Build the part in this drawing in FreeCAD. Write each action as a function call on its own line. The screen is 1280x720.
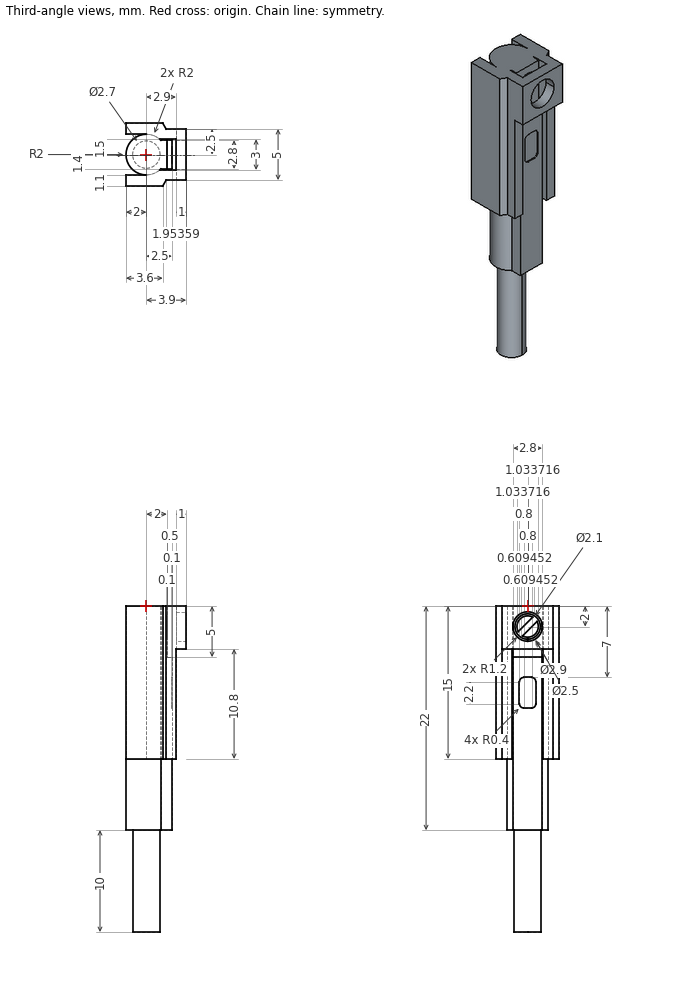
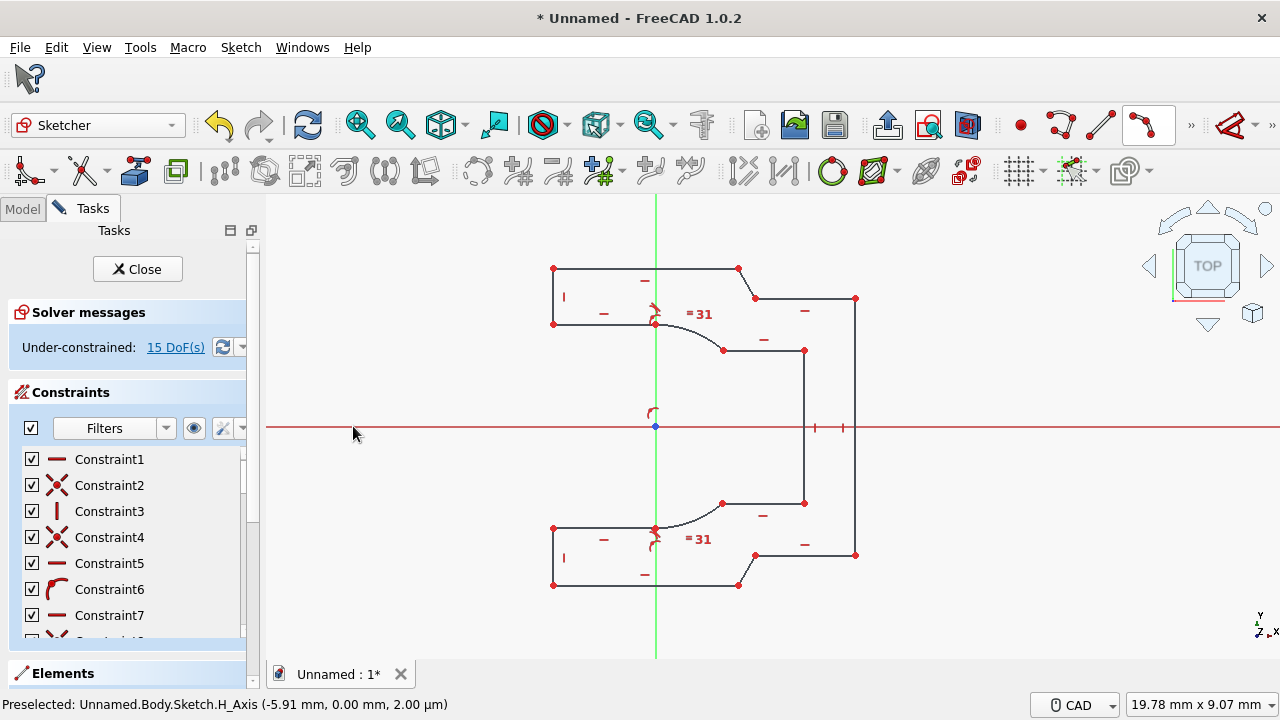
click(755, 556)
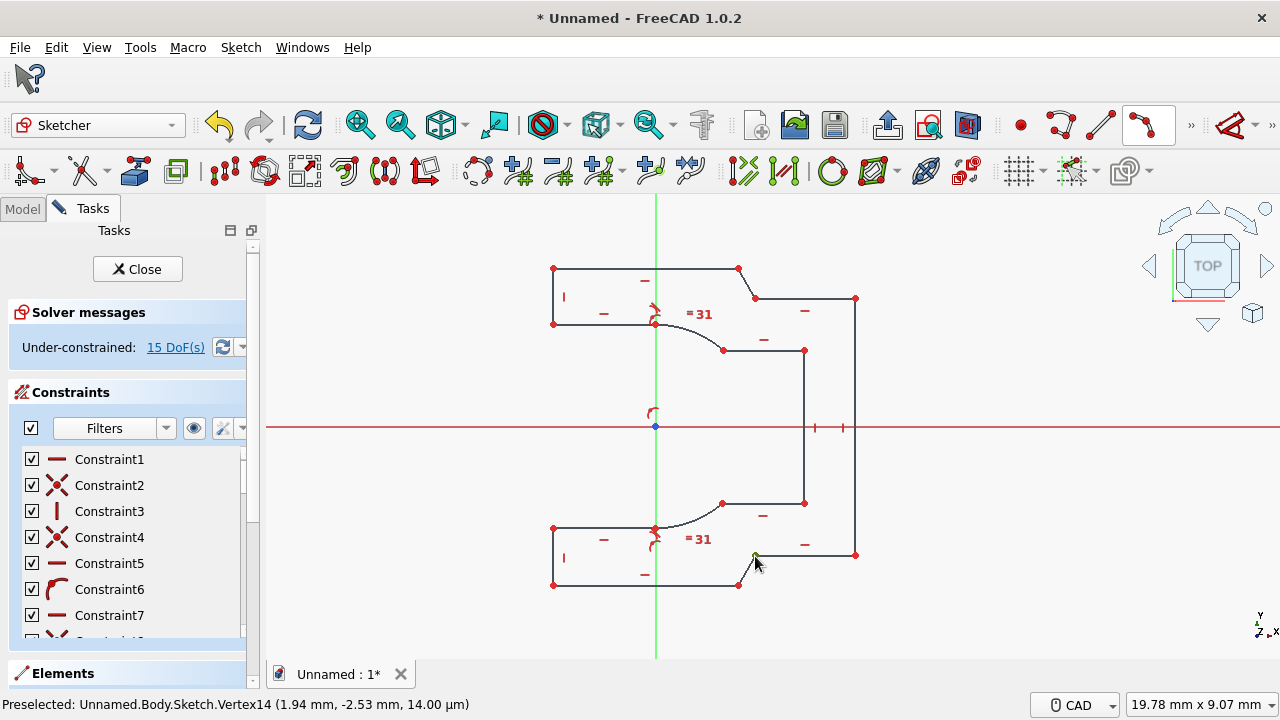
click(755, 299)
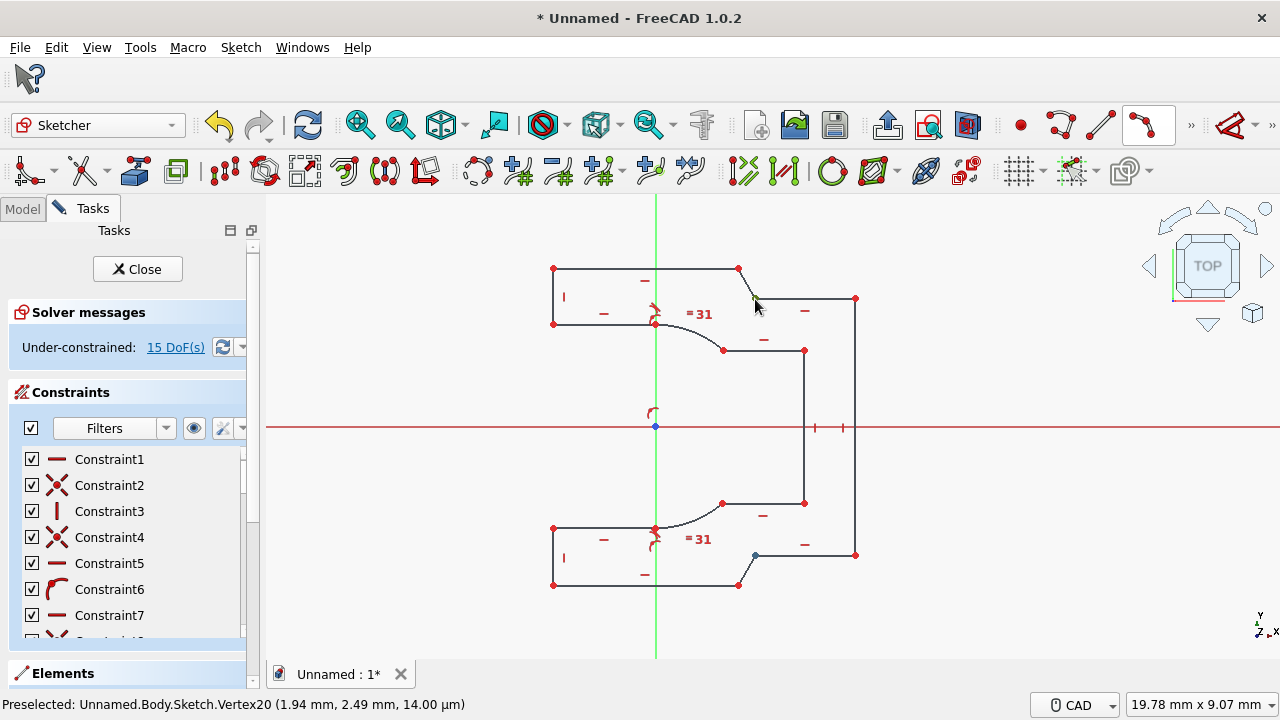
click(353, 426)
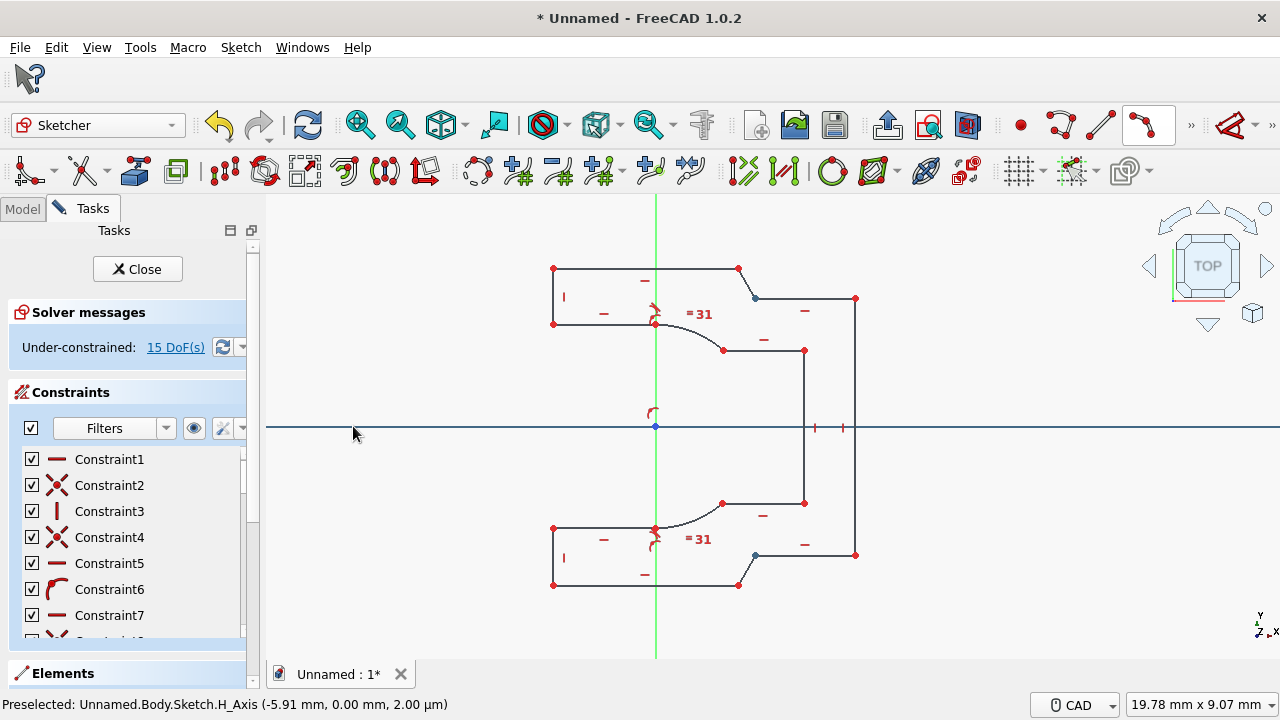
key(s)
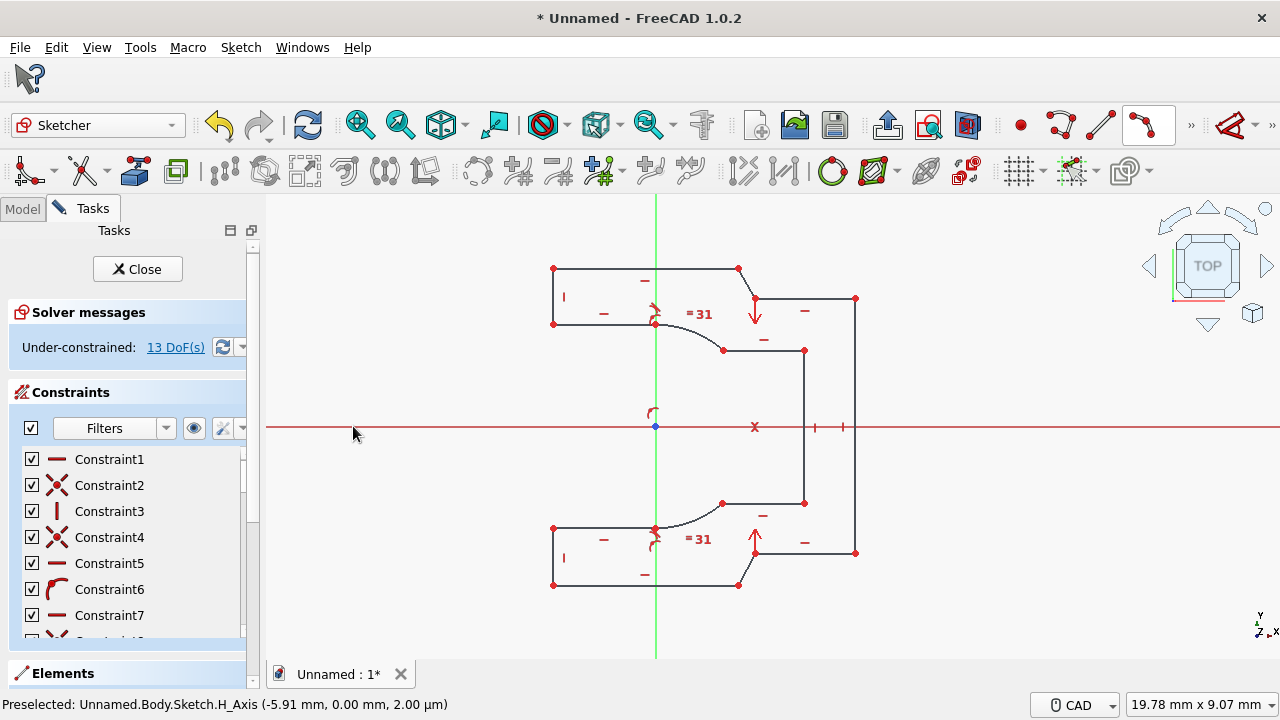
click(738, 586)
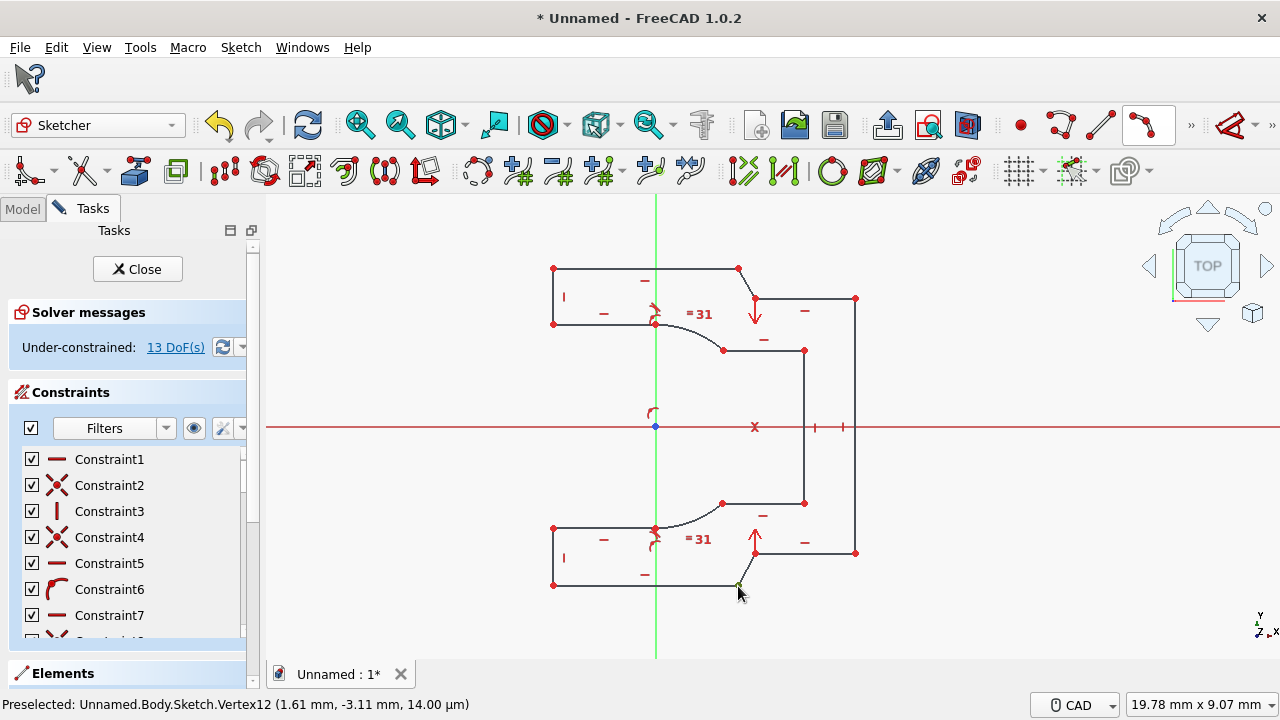
click(738, 269)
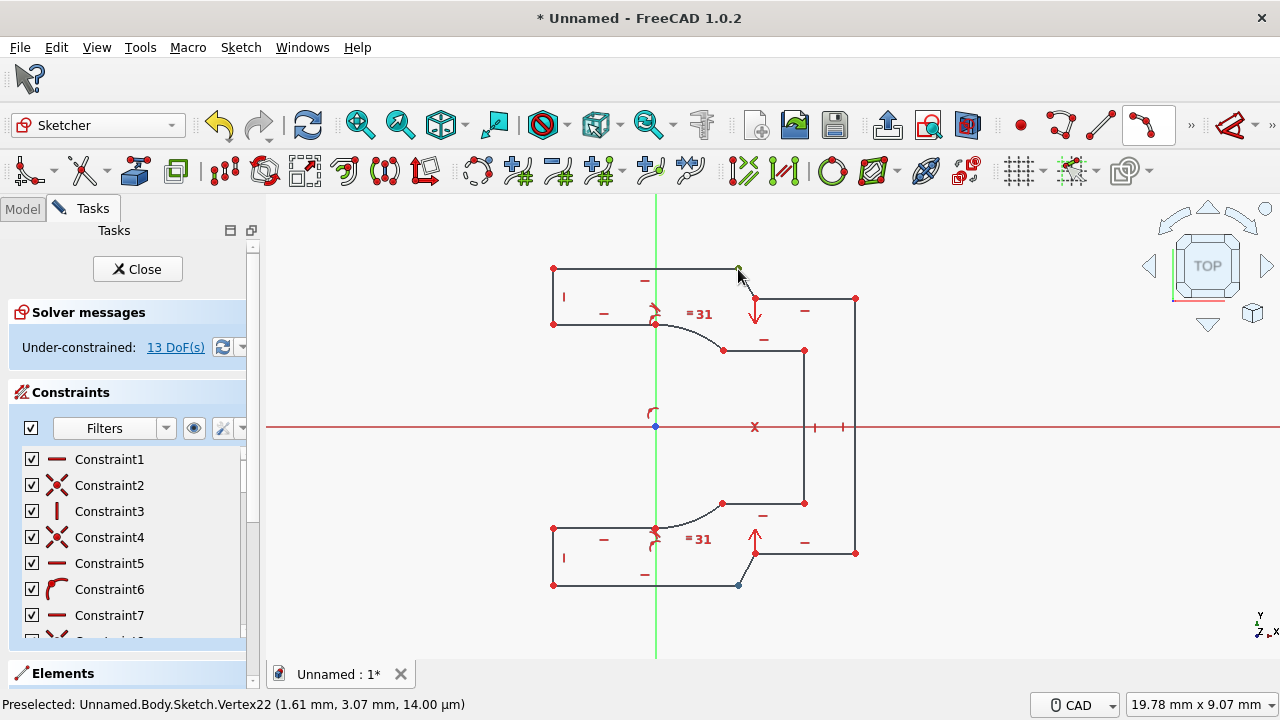
click(353, 426)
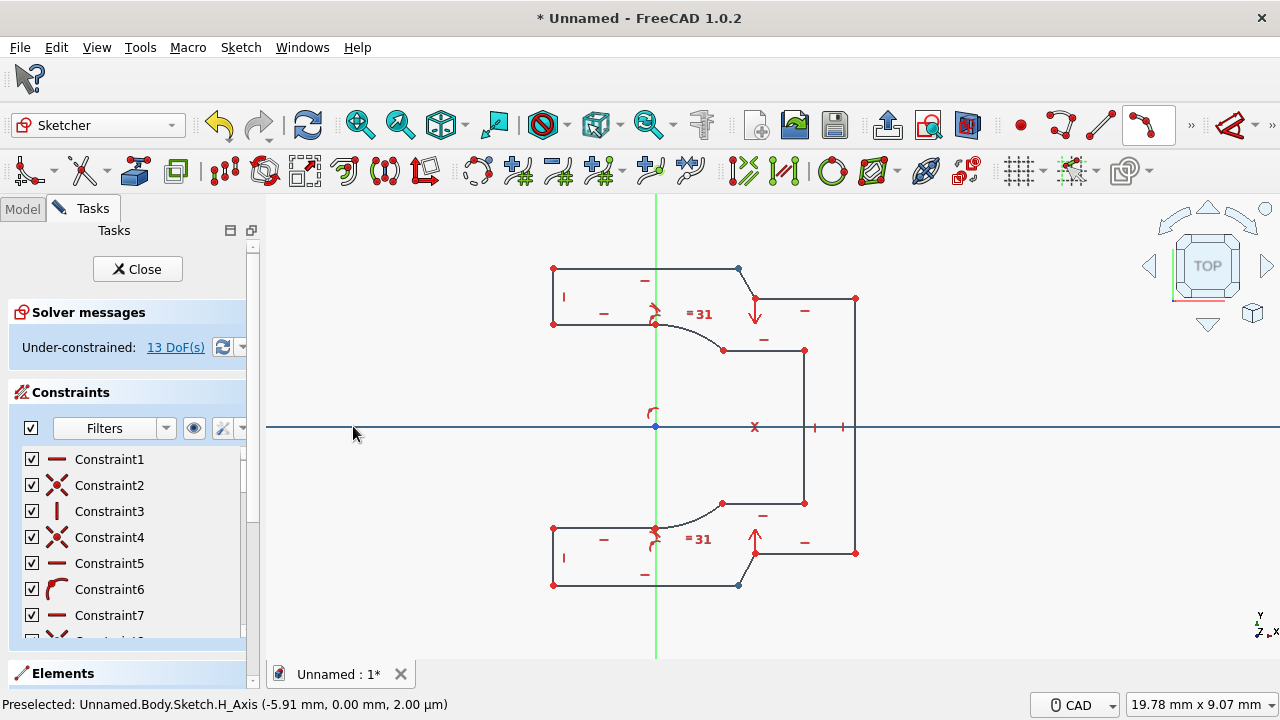
key(s)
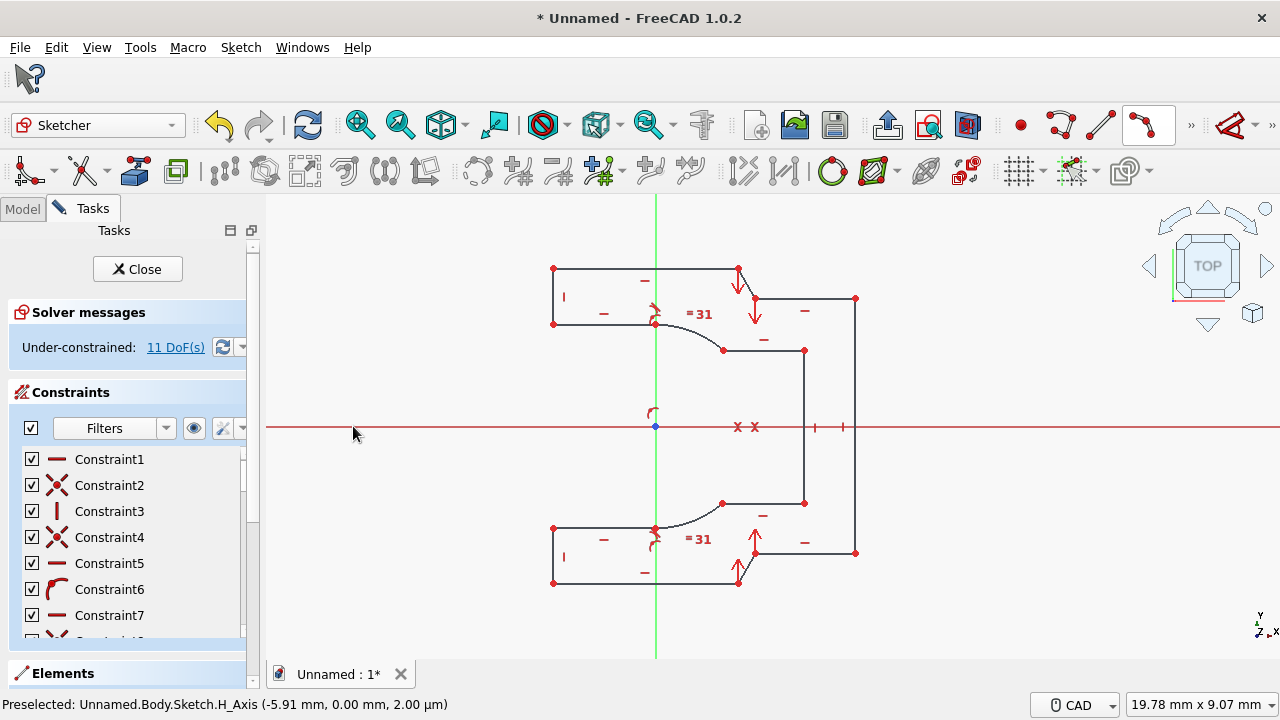
click(1230, 126)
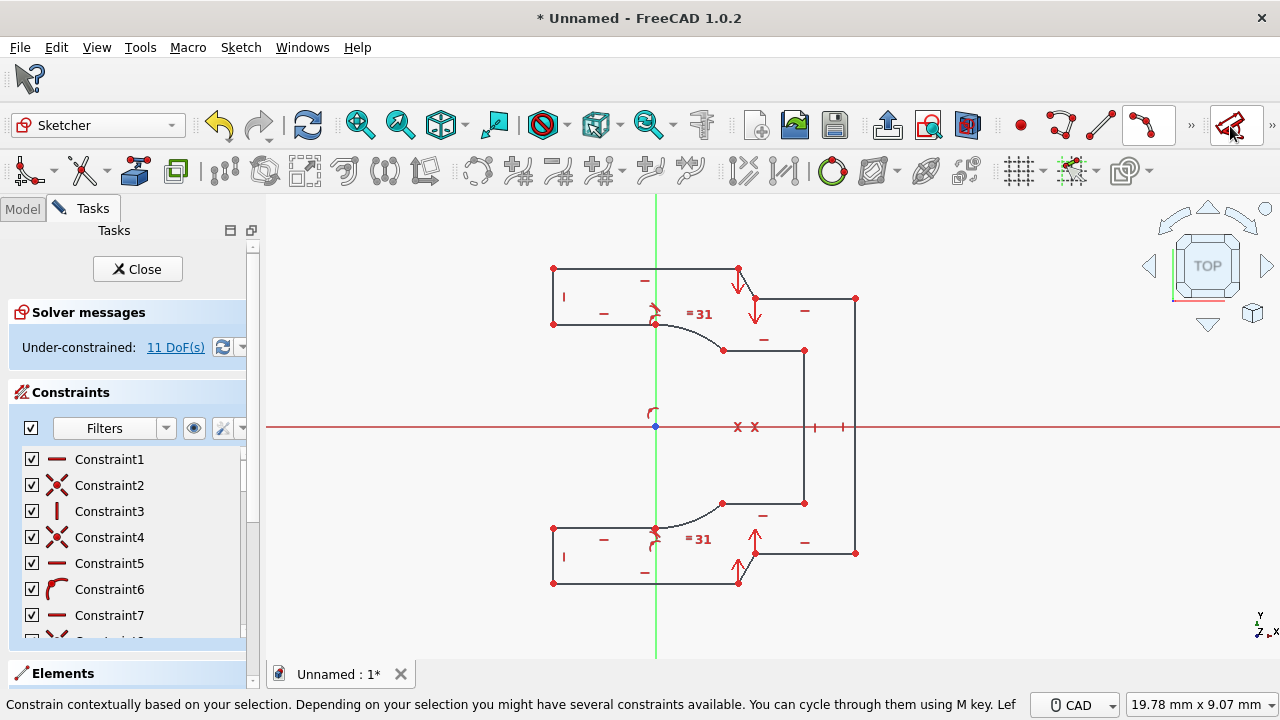
click(677, 526)
click(684, 557)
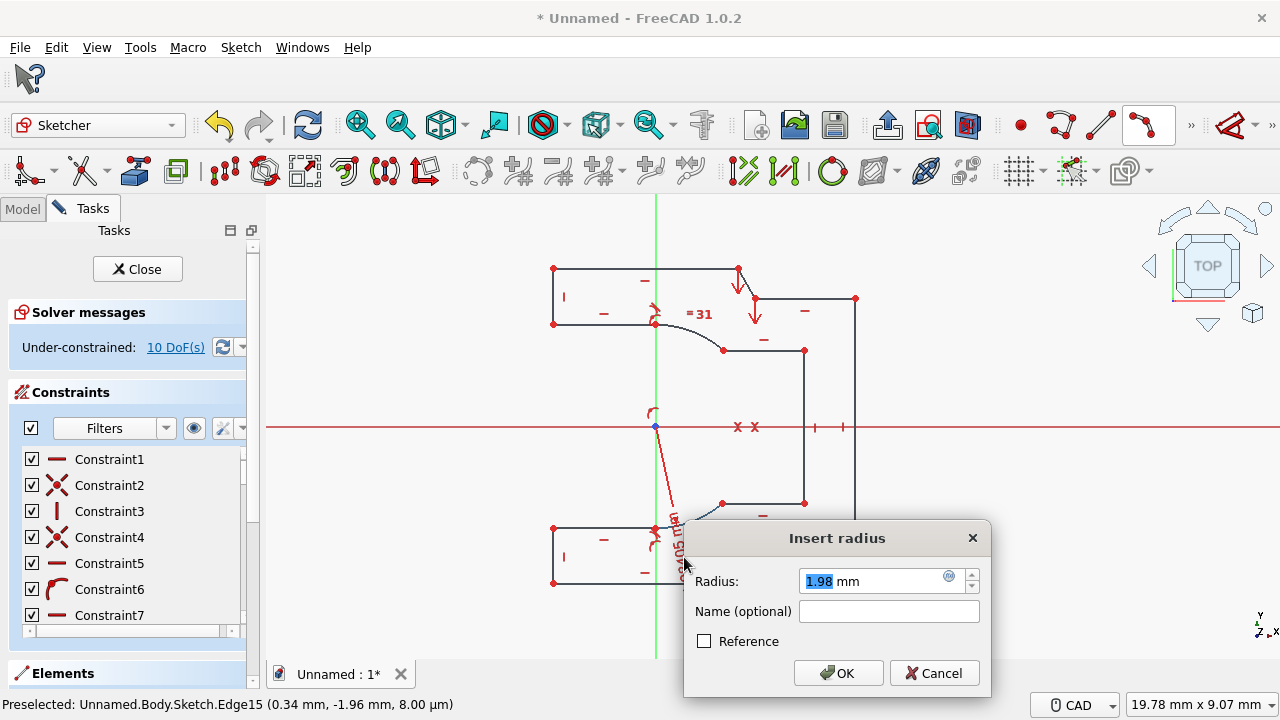
text(2)
key(Return)